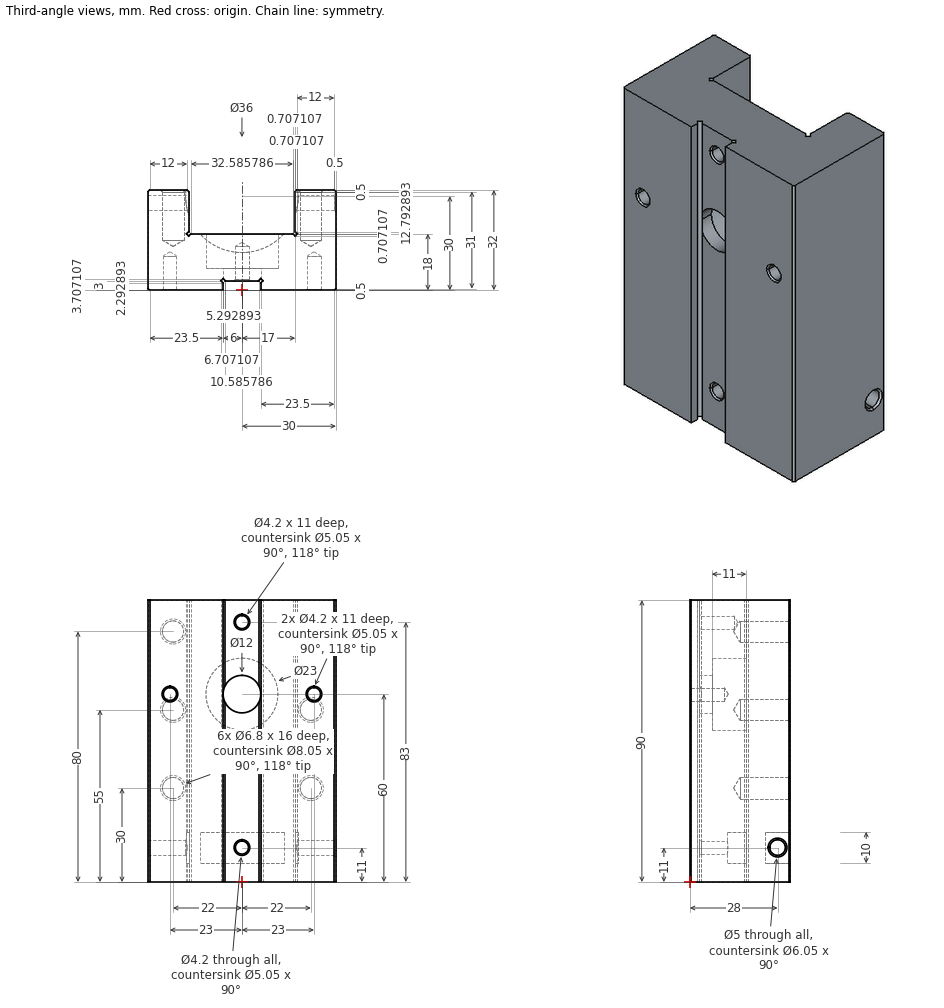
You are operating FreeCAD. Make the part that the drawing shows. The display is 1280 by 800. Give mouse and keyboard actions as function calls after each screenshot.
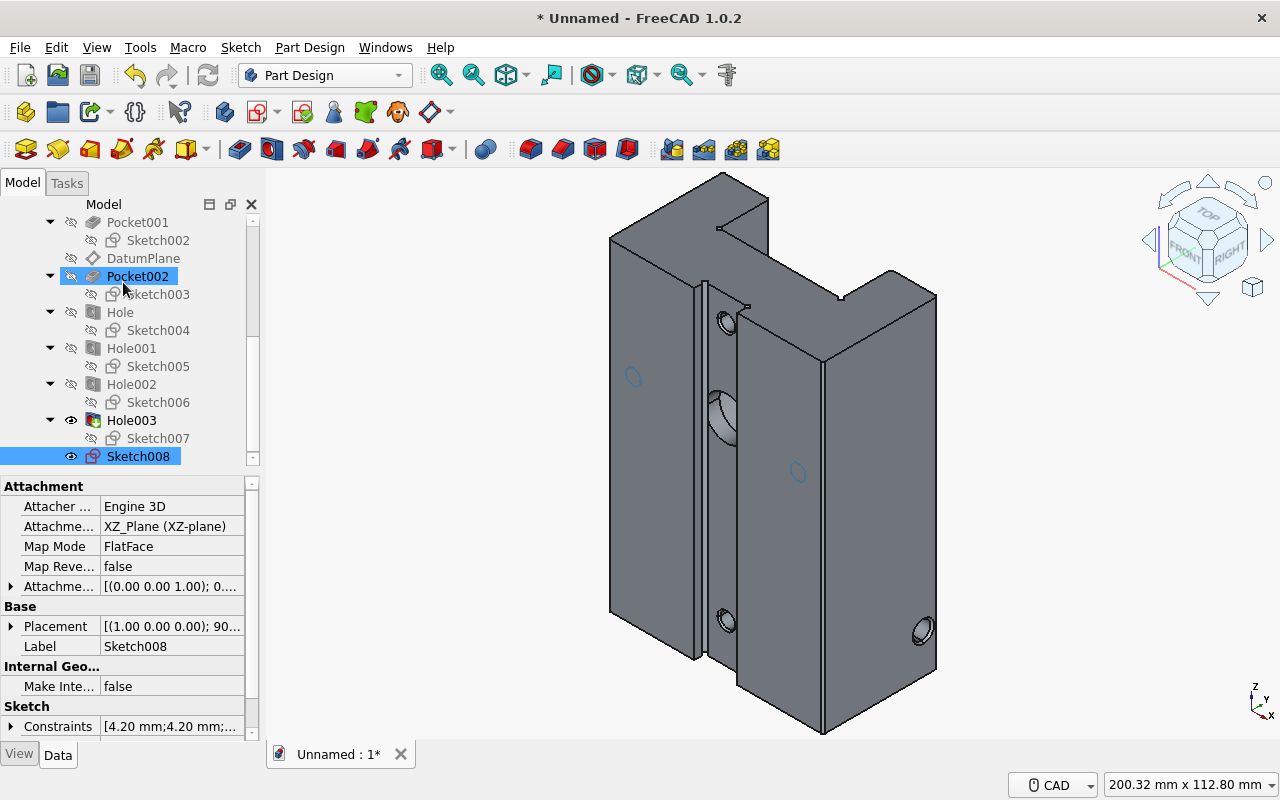
click(272, 150)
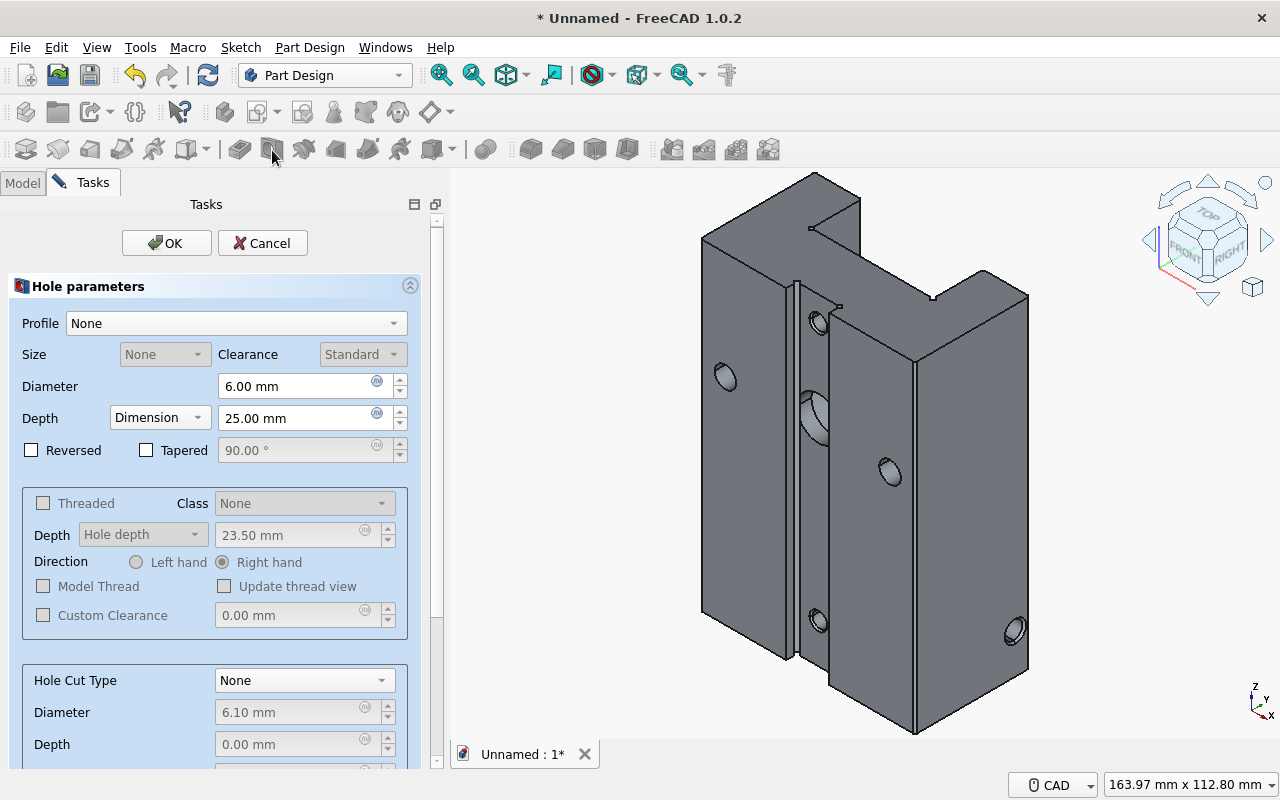
triple_click(305, 386)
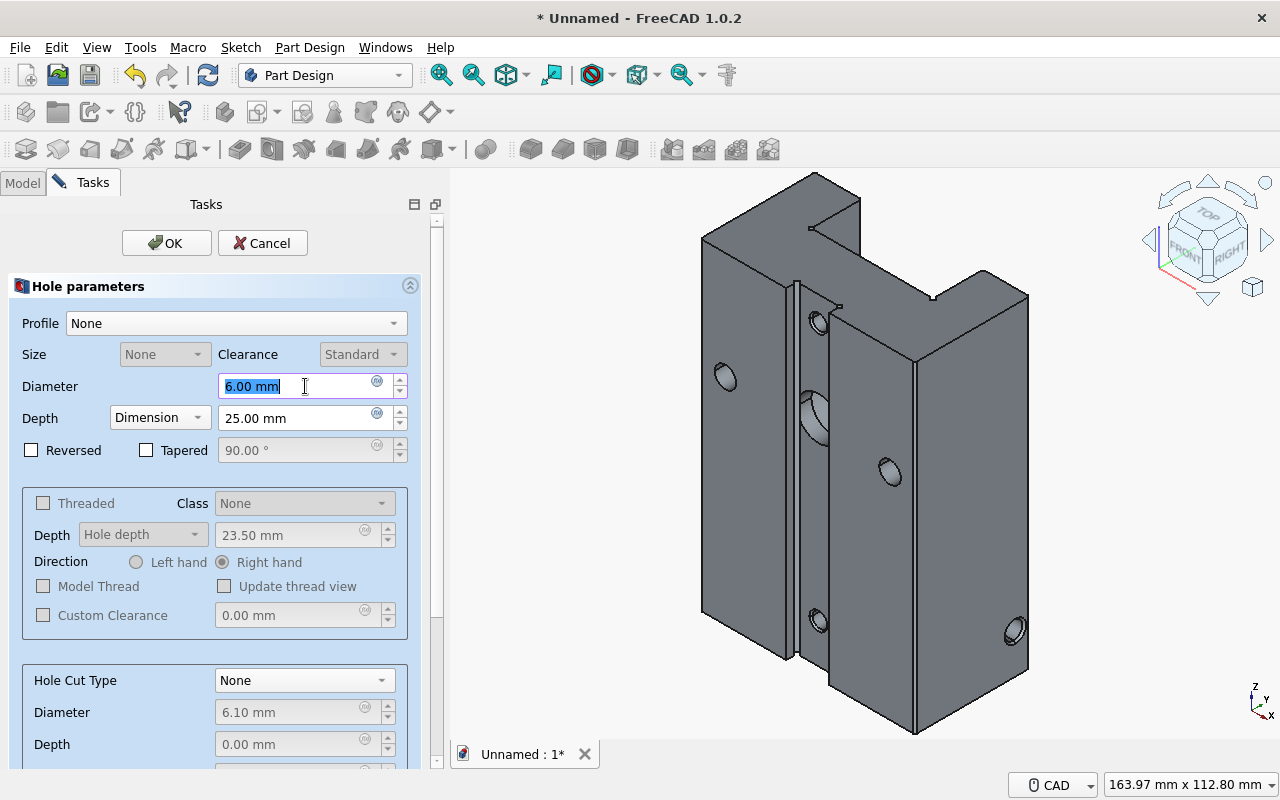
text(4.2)
key(Tab)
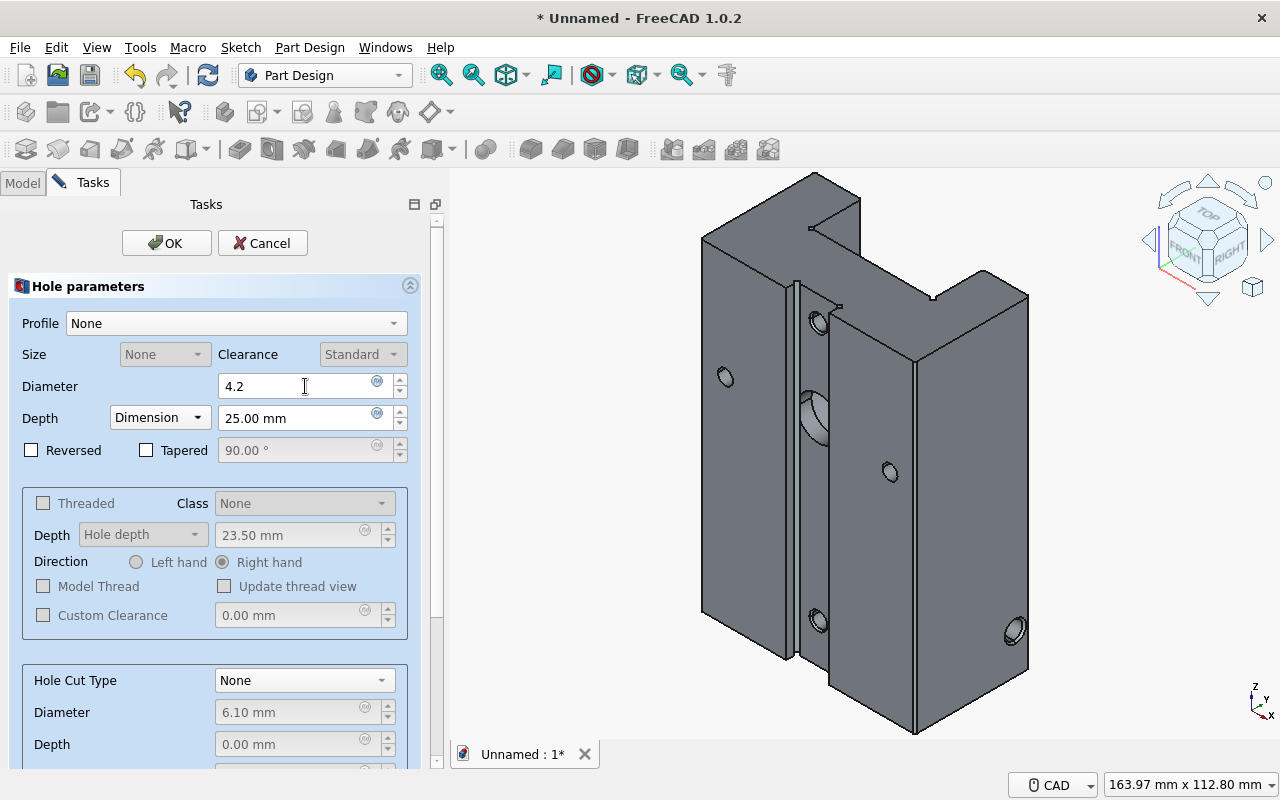
triple_click(305, 418)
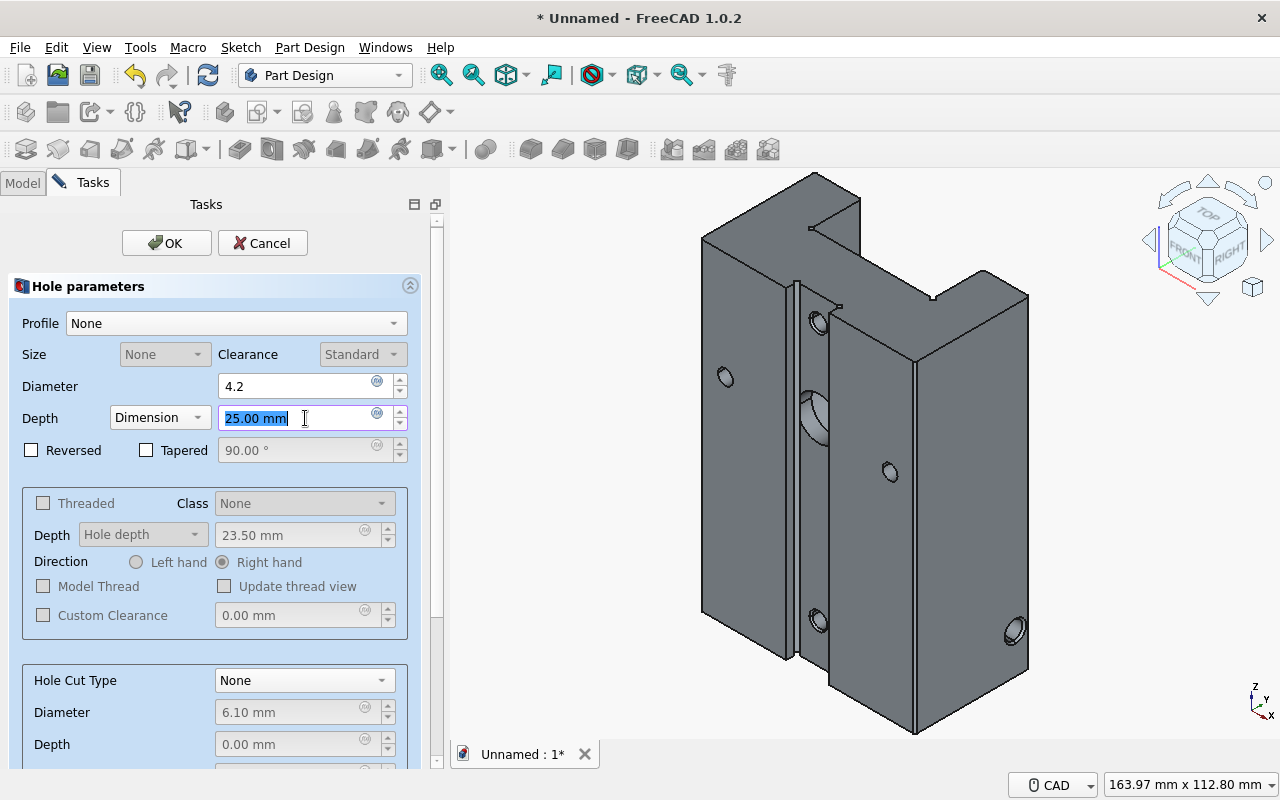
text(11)
key(Tab)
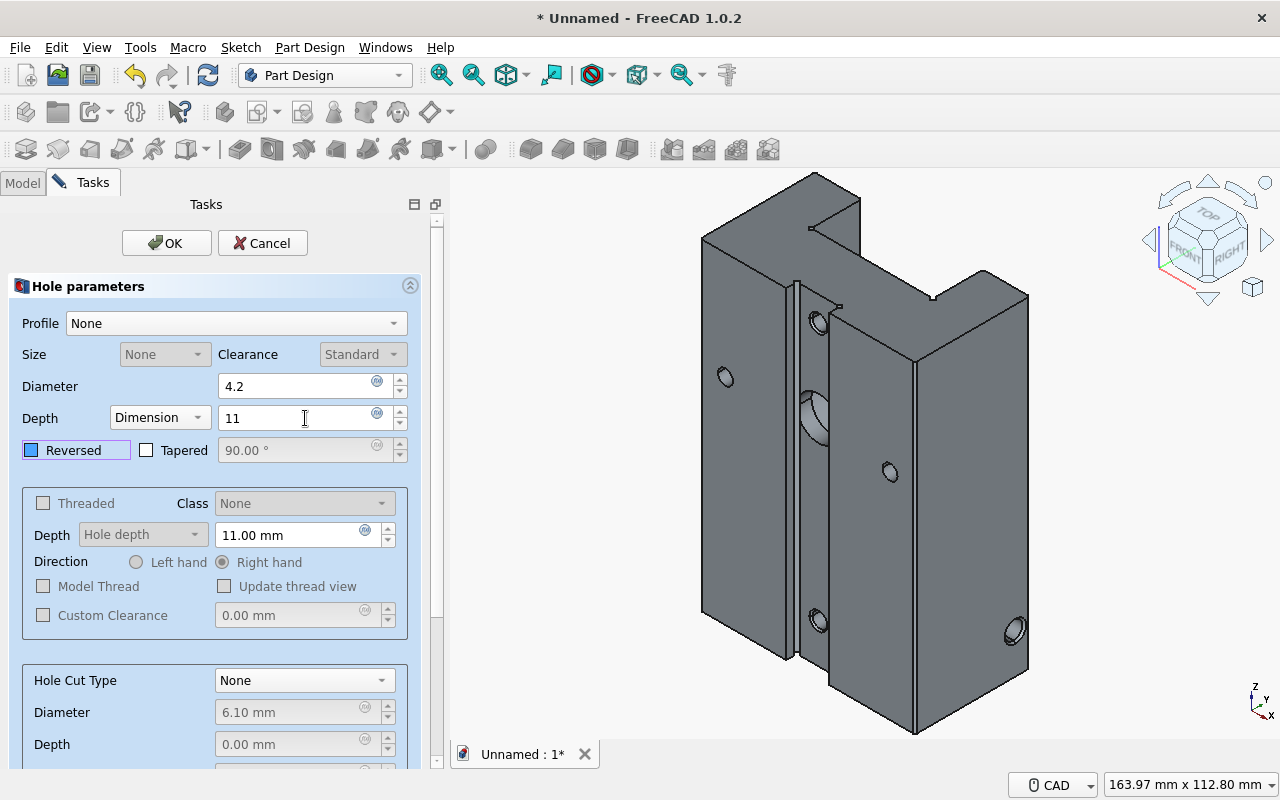
click(306, 680)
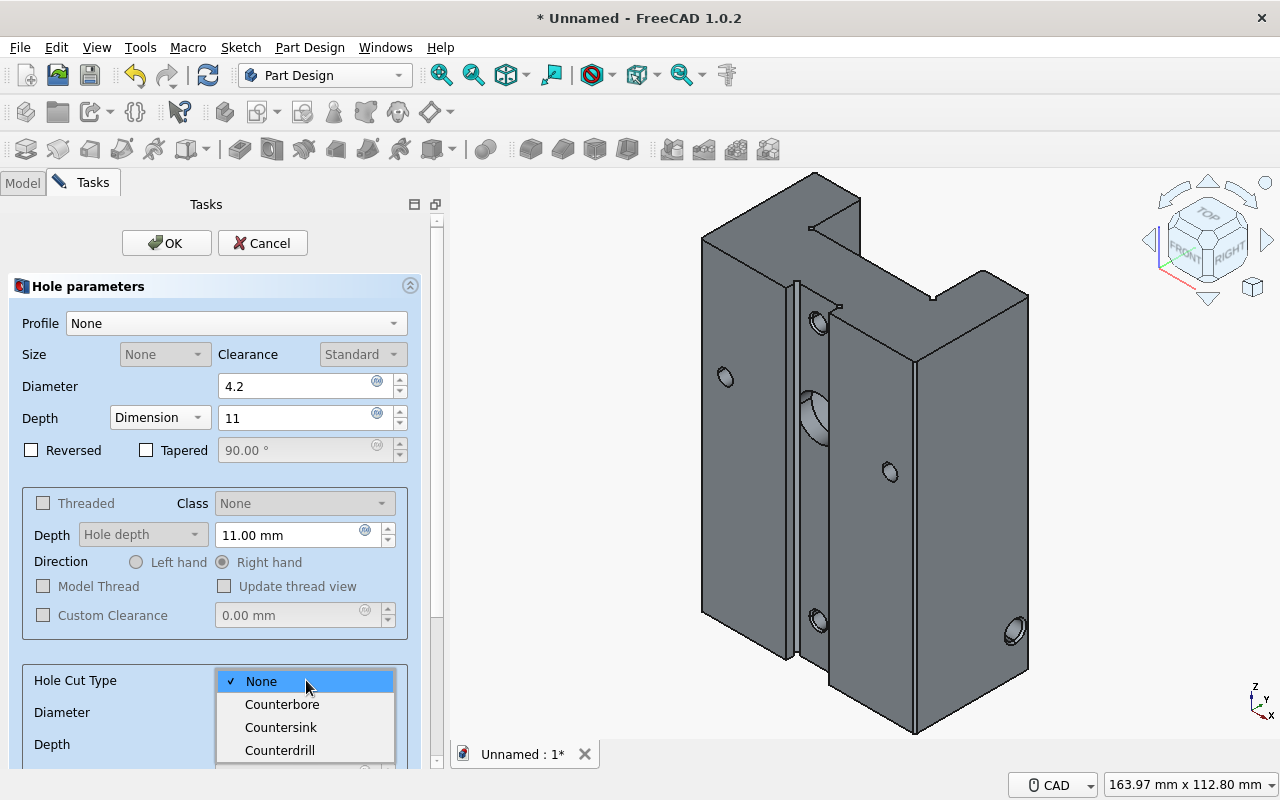
click(304, 728)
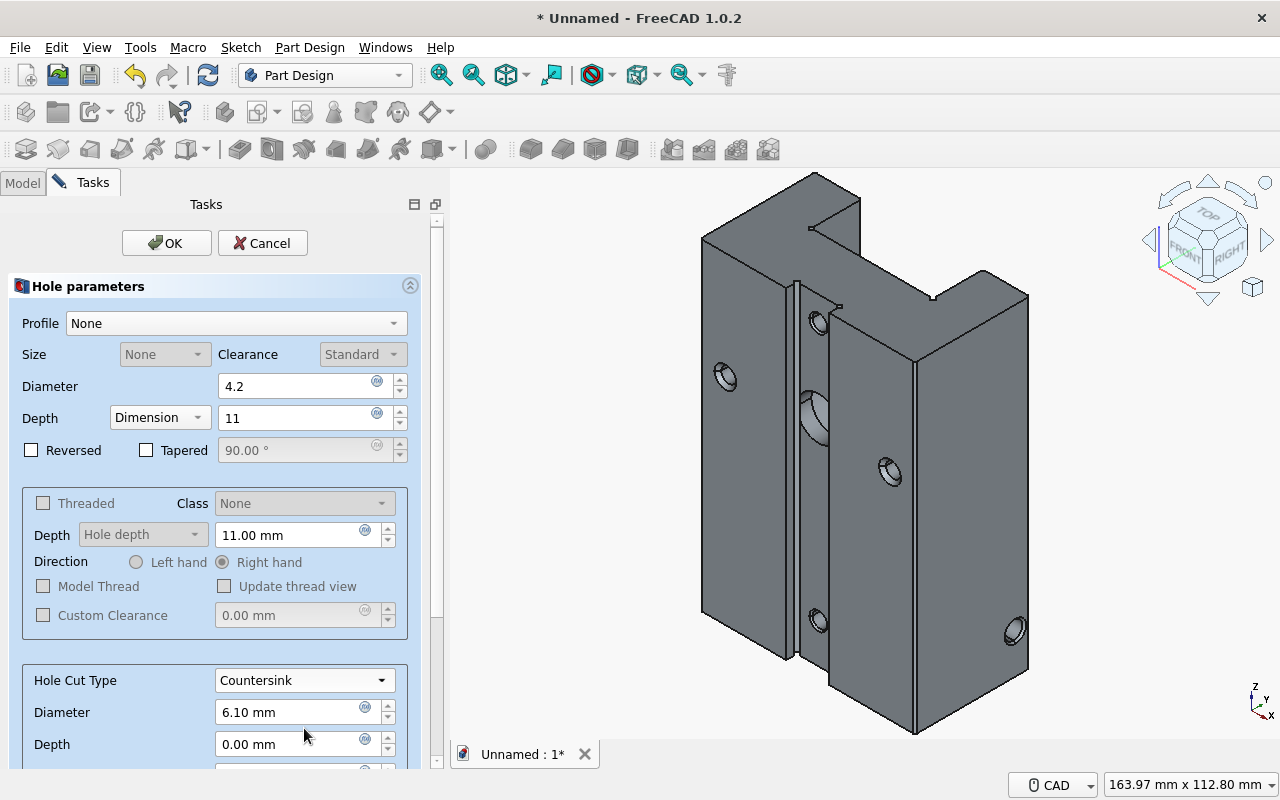
triple_click(298, 712)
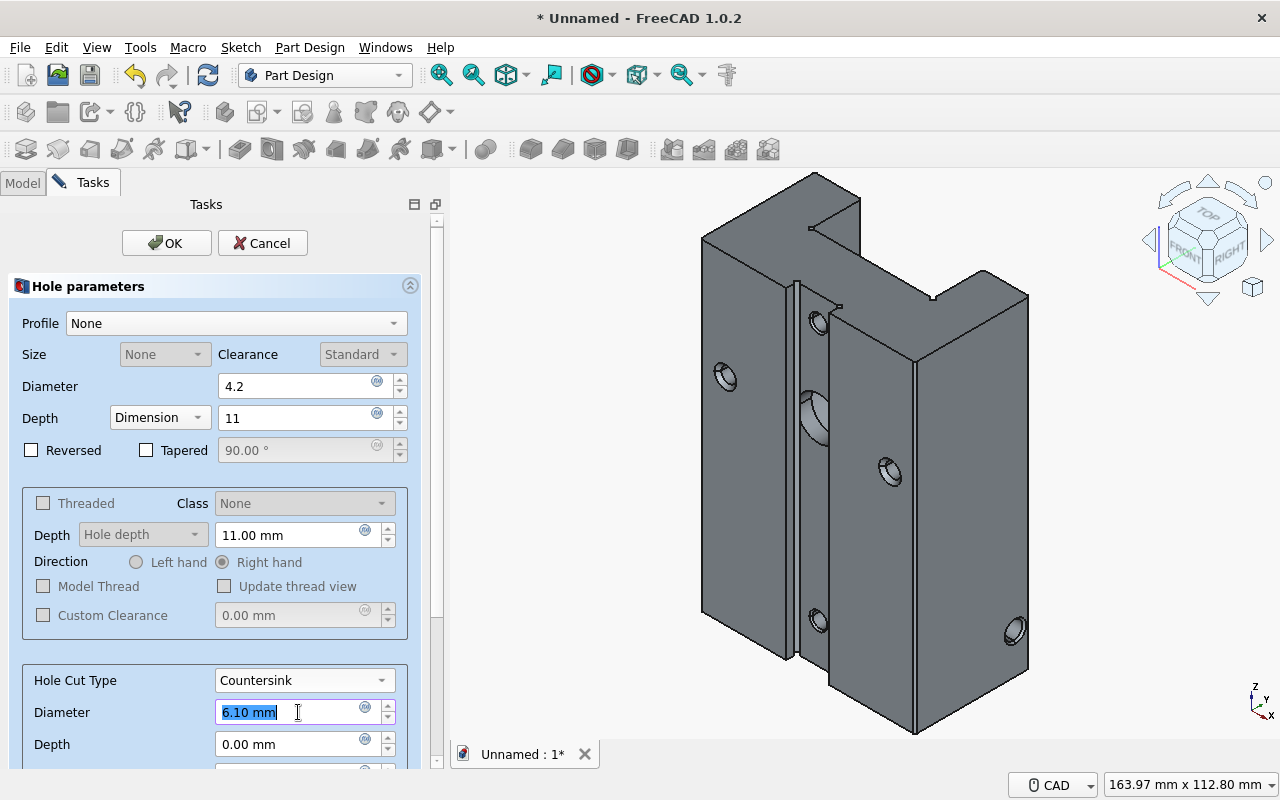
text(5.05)
key(Tab)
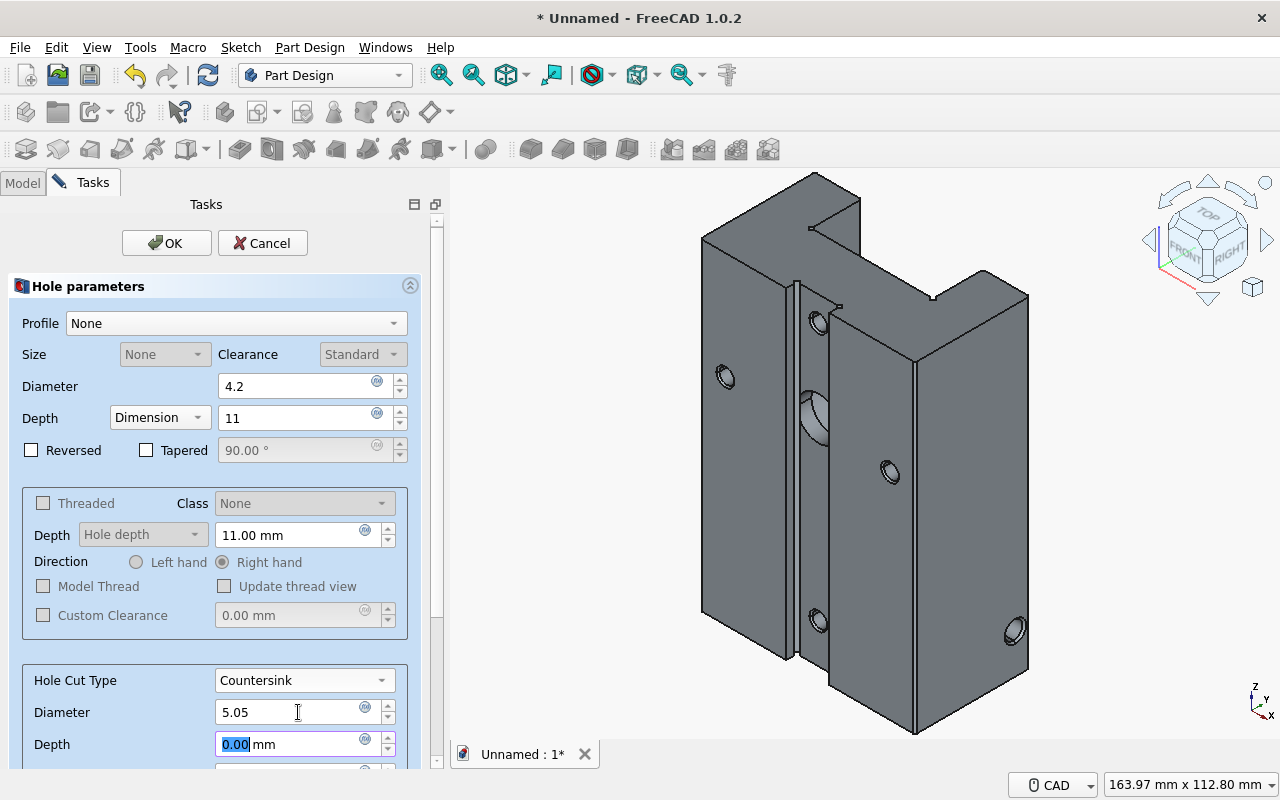
click(167, 243)